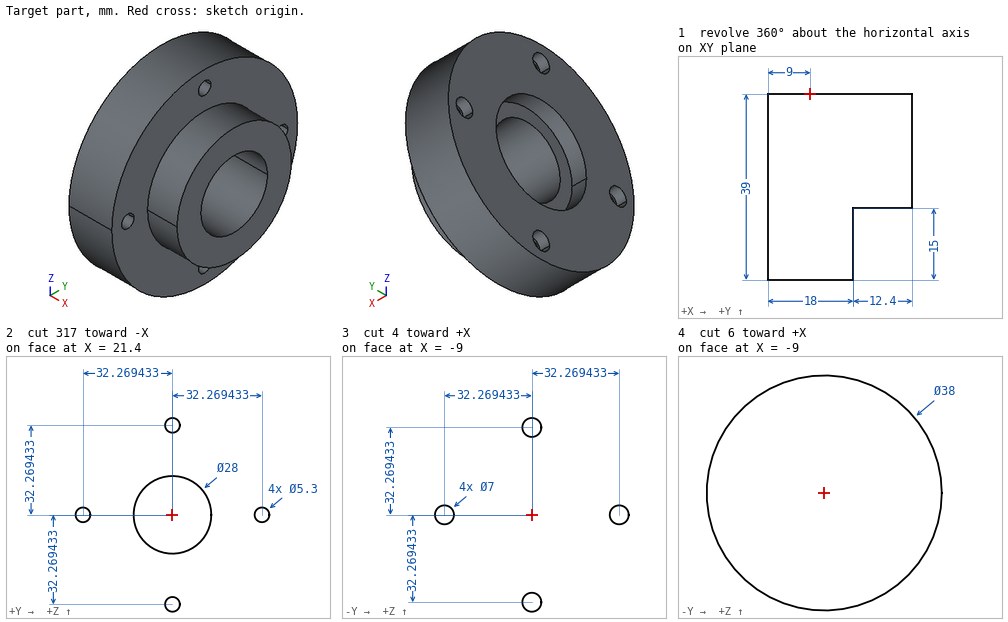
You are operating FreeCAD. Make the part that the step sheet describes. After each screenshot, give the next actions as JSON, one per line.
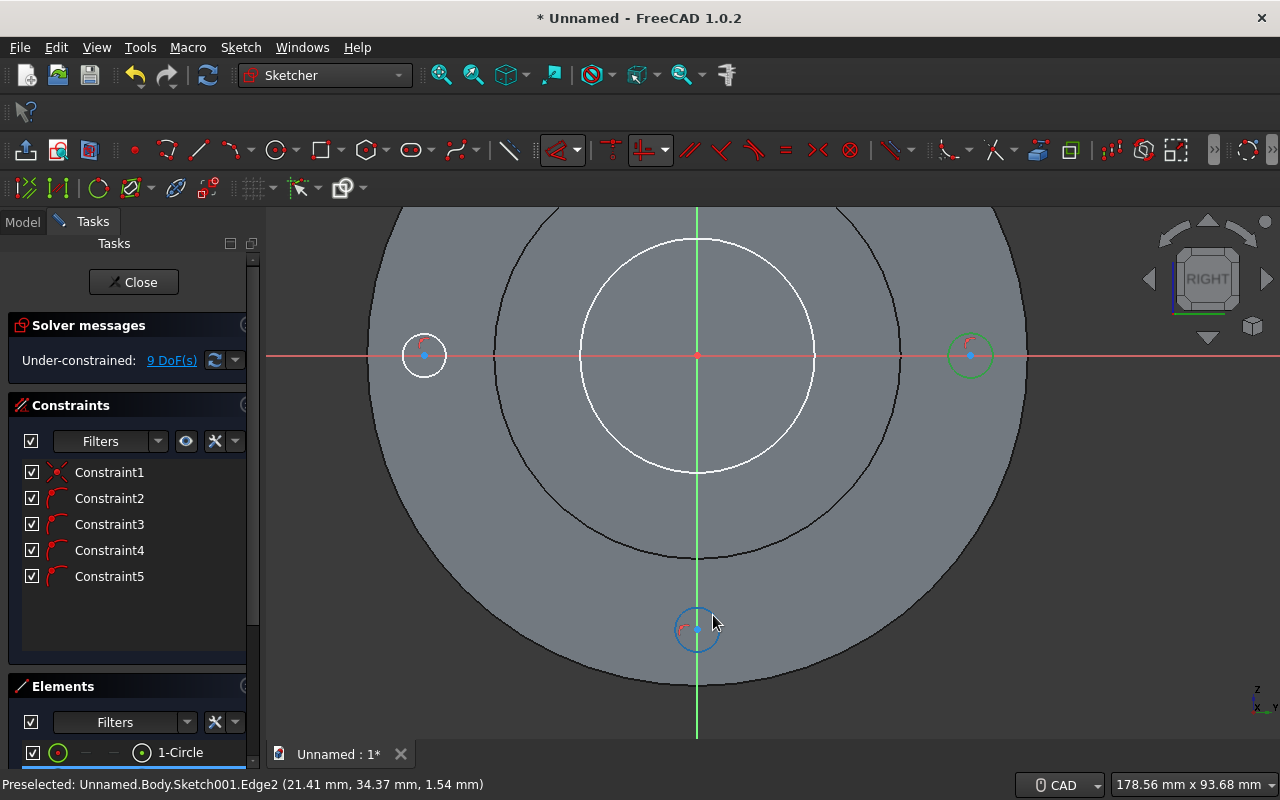
{"action": "left_click", "coordinate": [713, 614]}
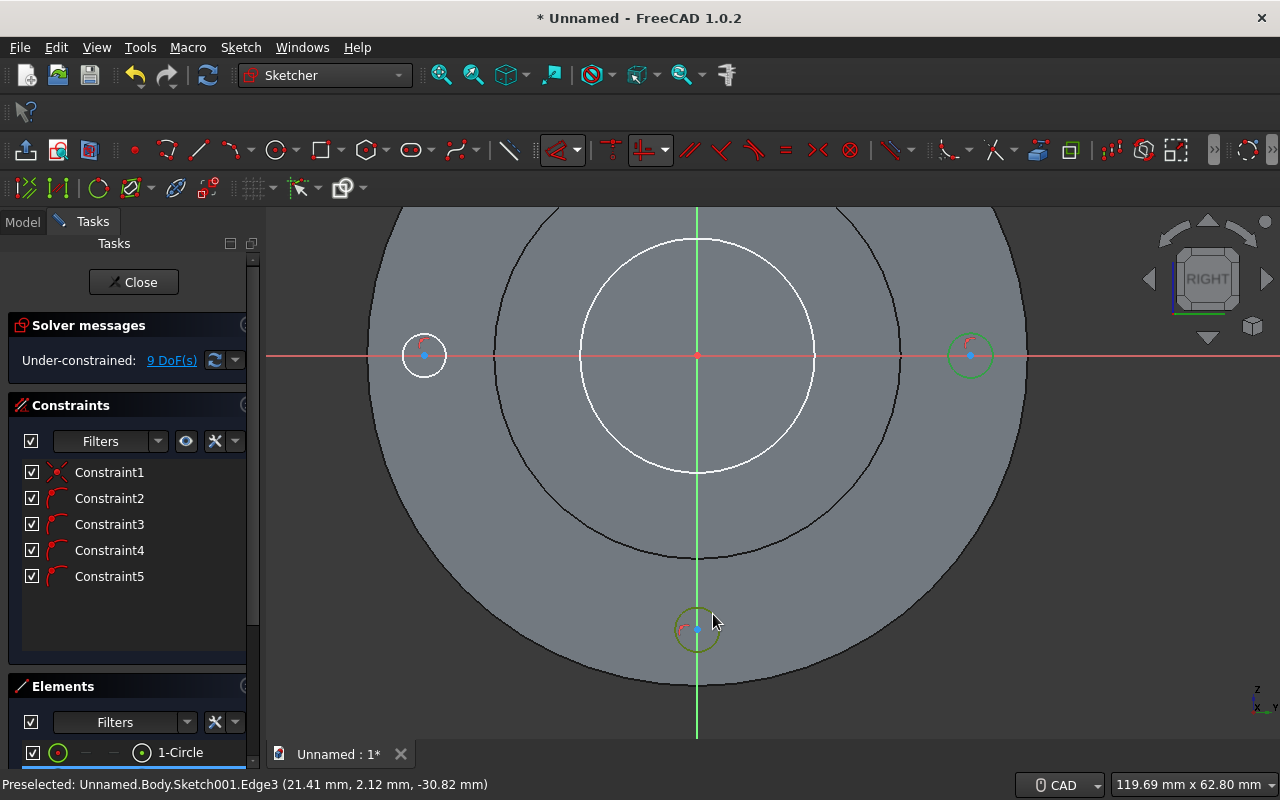
{"action": "left_click", "coordinate": [439, 340]}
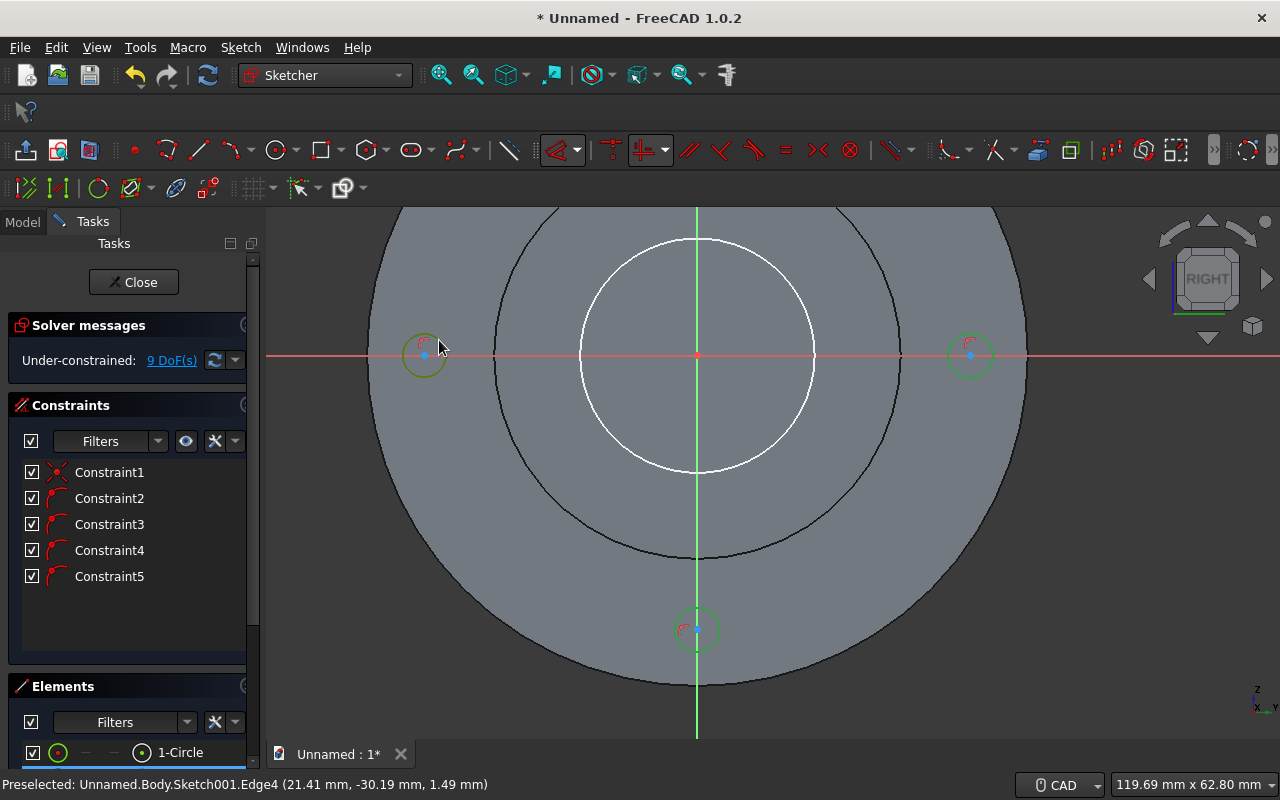
{"action": "scroll", "coordinate": [713, 616], "scroll_direction": "down", "scroll_amount": 3}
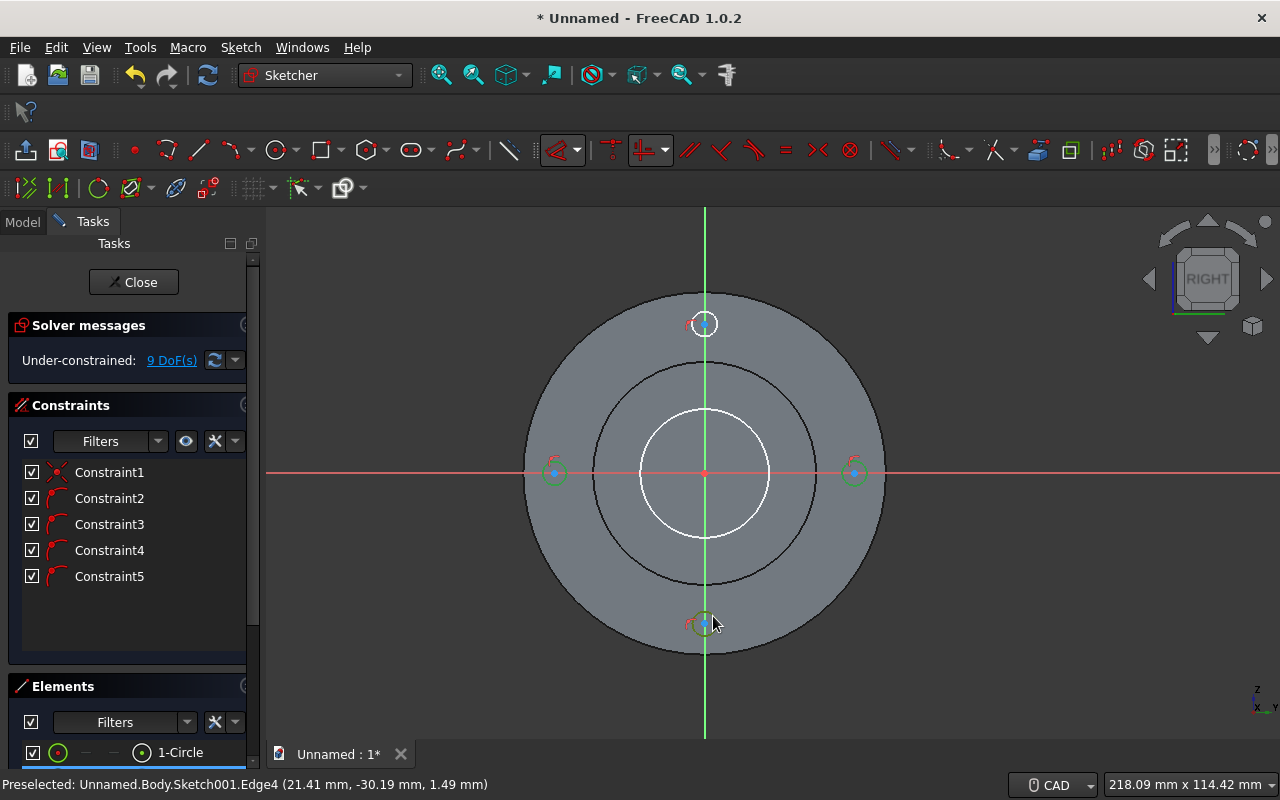
{"action": "scroll", "coordinate": [713, 315], "scroll_direction": "up", "scroll_amount": 3}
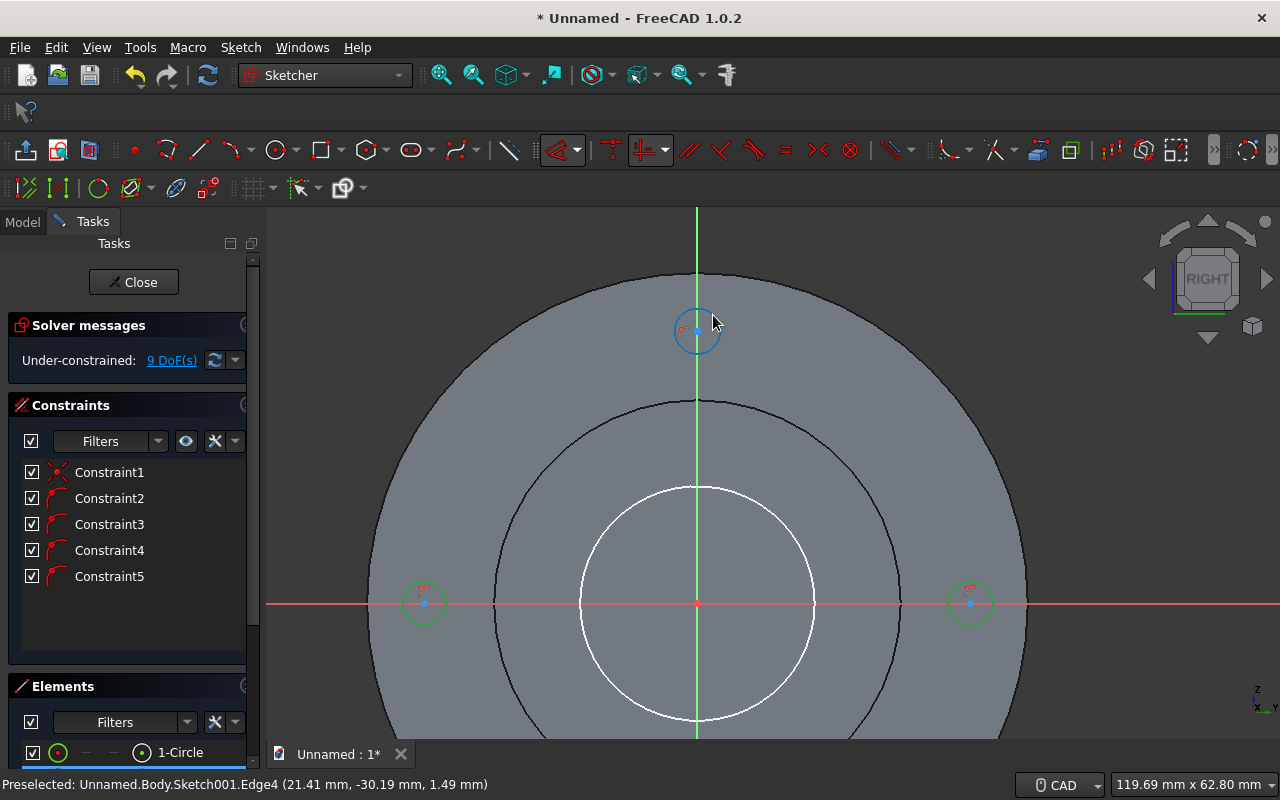
{"action": "left_click", "coordinate": [713, 315]}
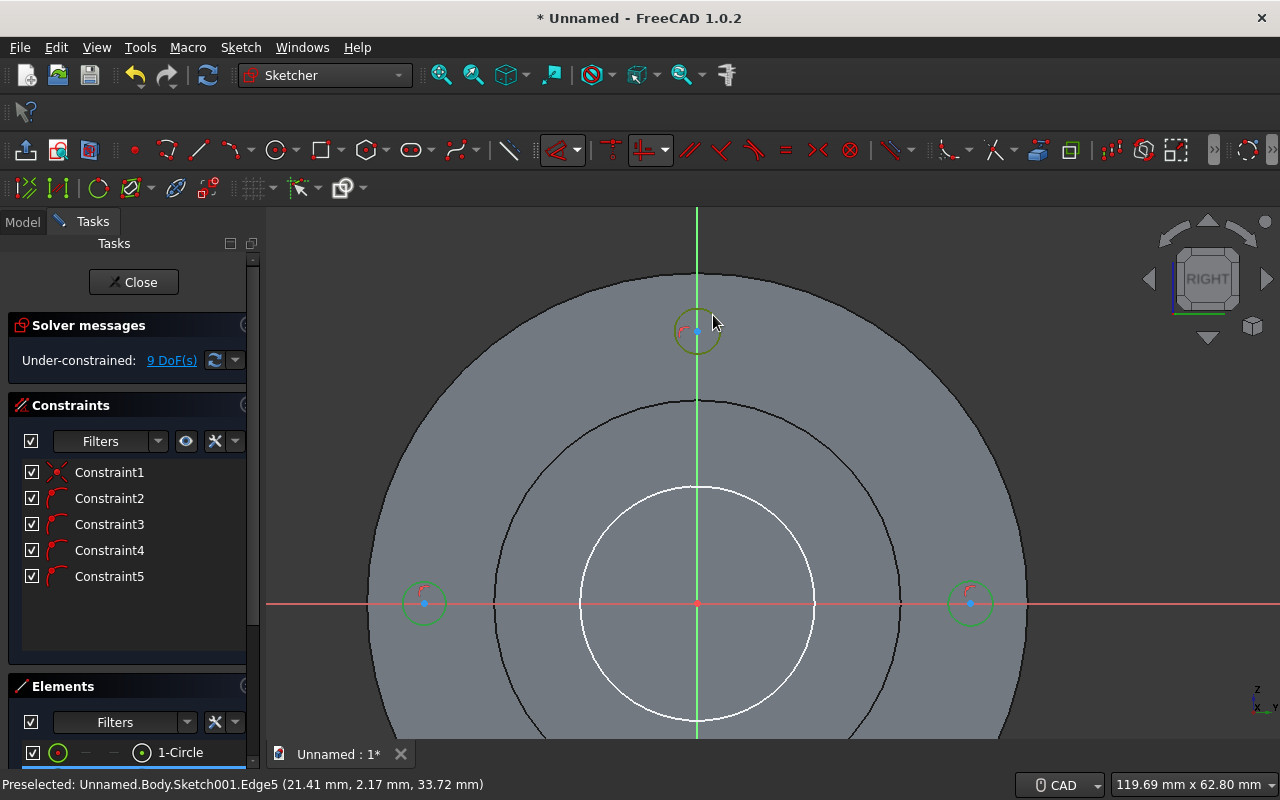
{"action": "left_click", "coordinate": [786, 150]}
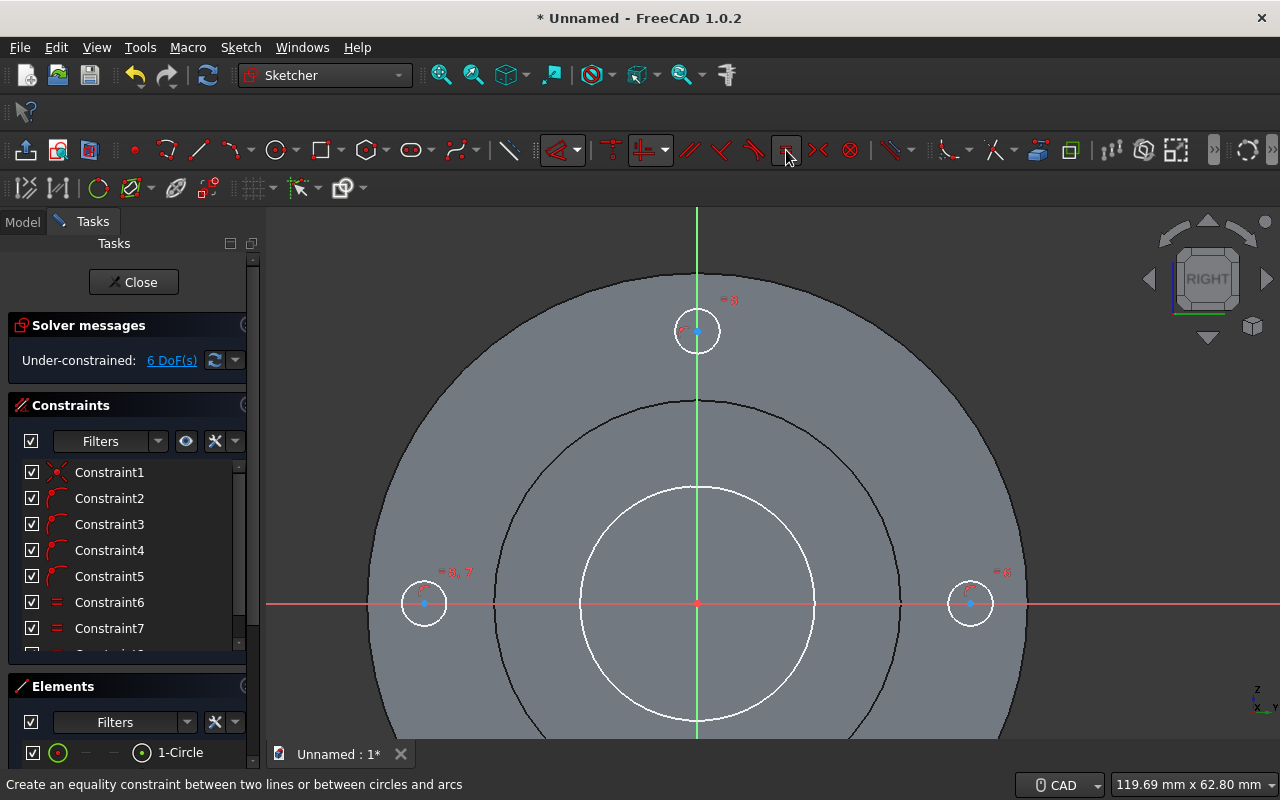
{"action": "left_click", "coordinate": [780, 520]}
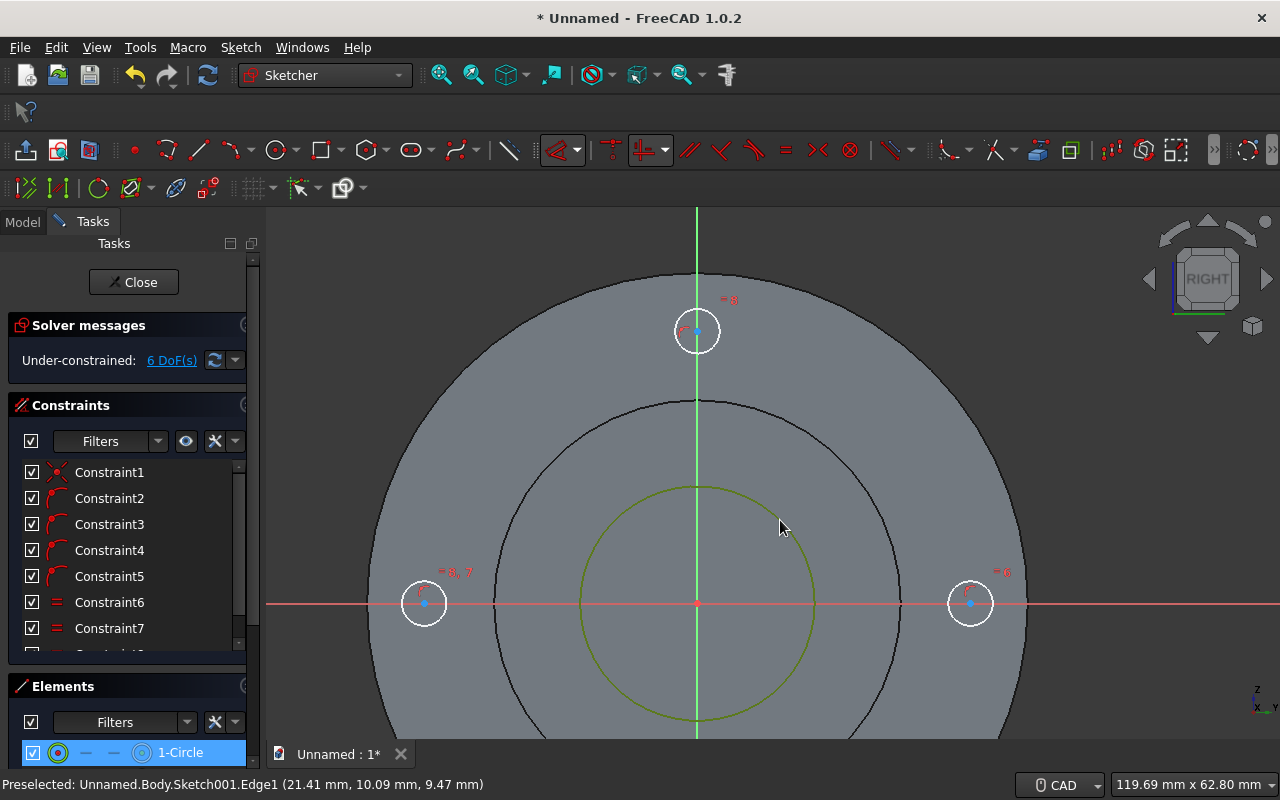
{"action": "key", "text": "k o"}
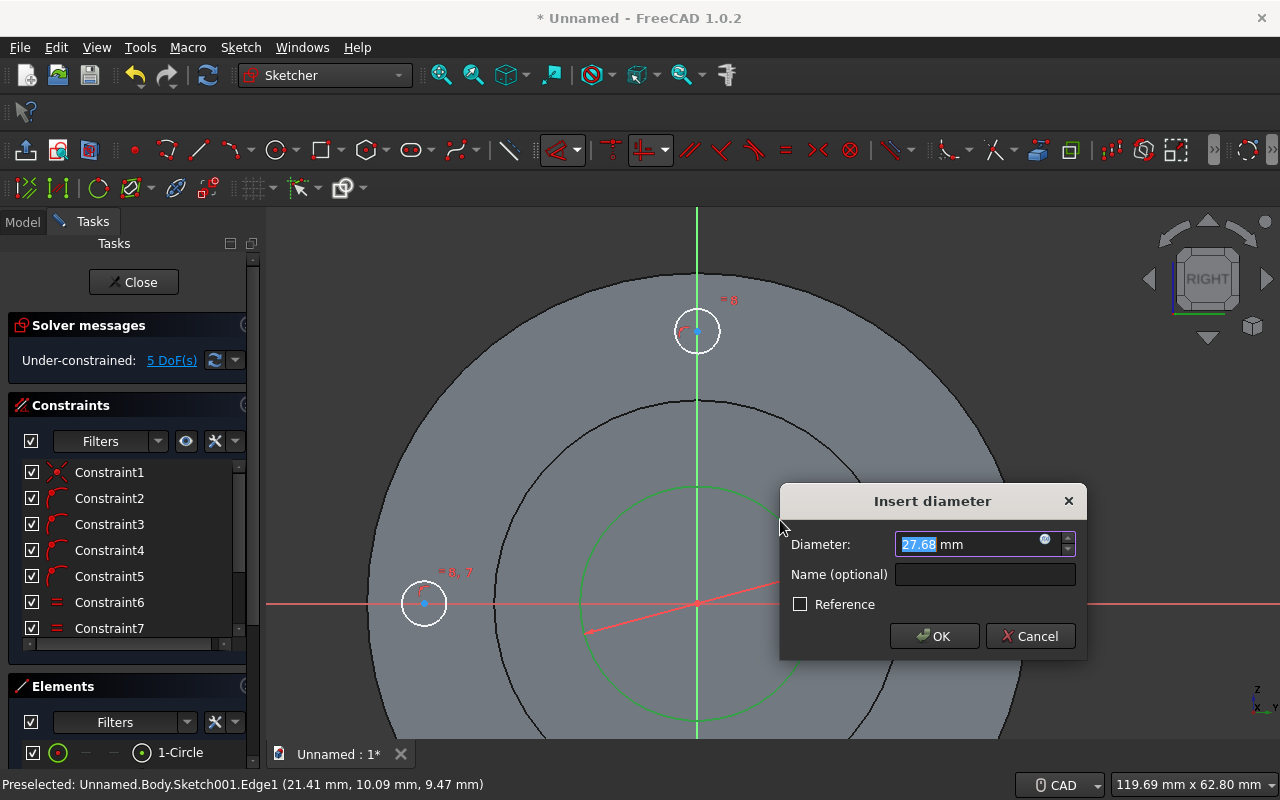
{"action": "type", "text": "28"}
{"action": "key", "text": "Return"}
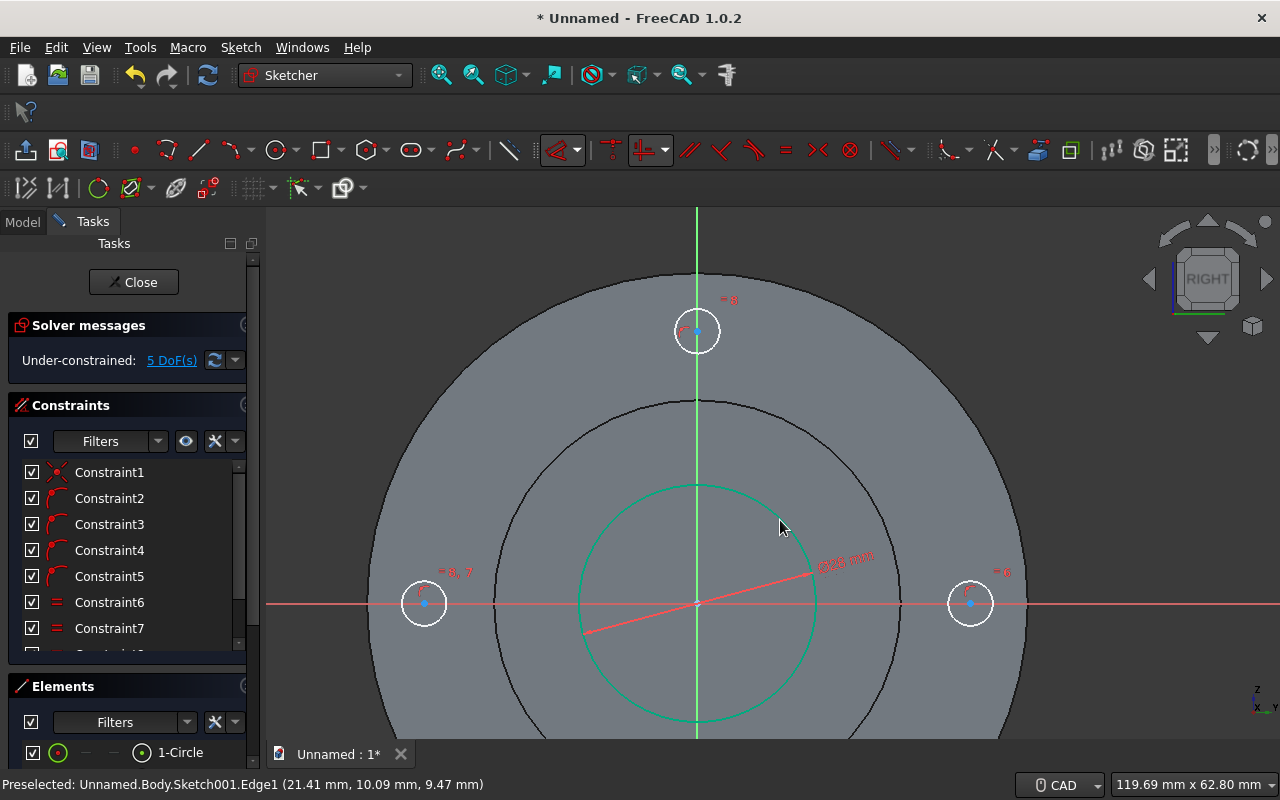
{"action": "left_click", "coordinate": [986, 588]}